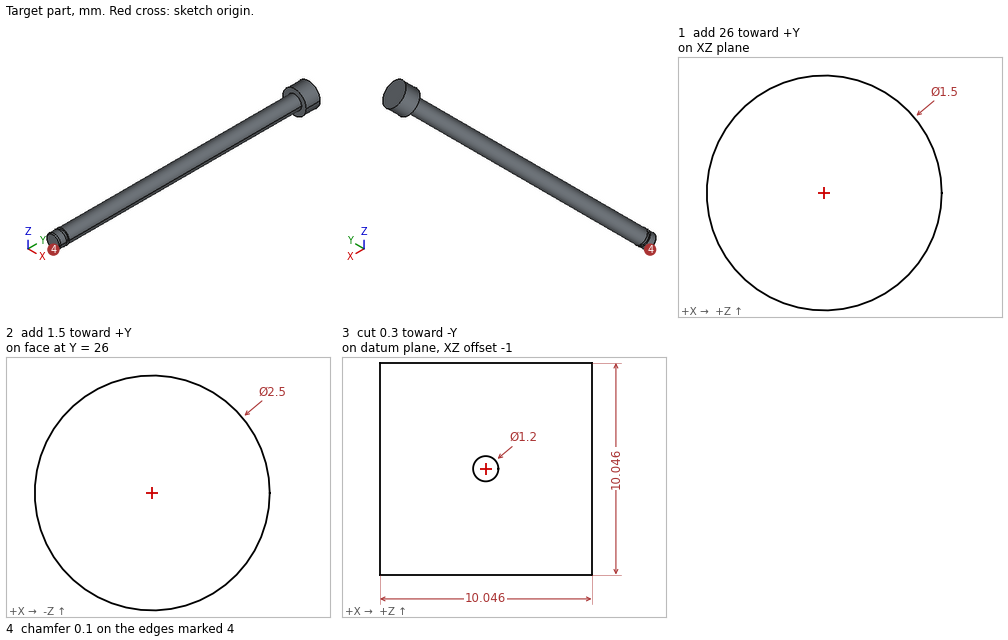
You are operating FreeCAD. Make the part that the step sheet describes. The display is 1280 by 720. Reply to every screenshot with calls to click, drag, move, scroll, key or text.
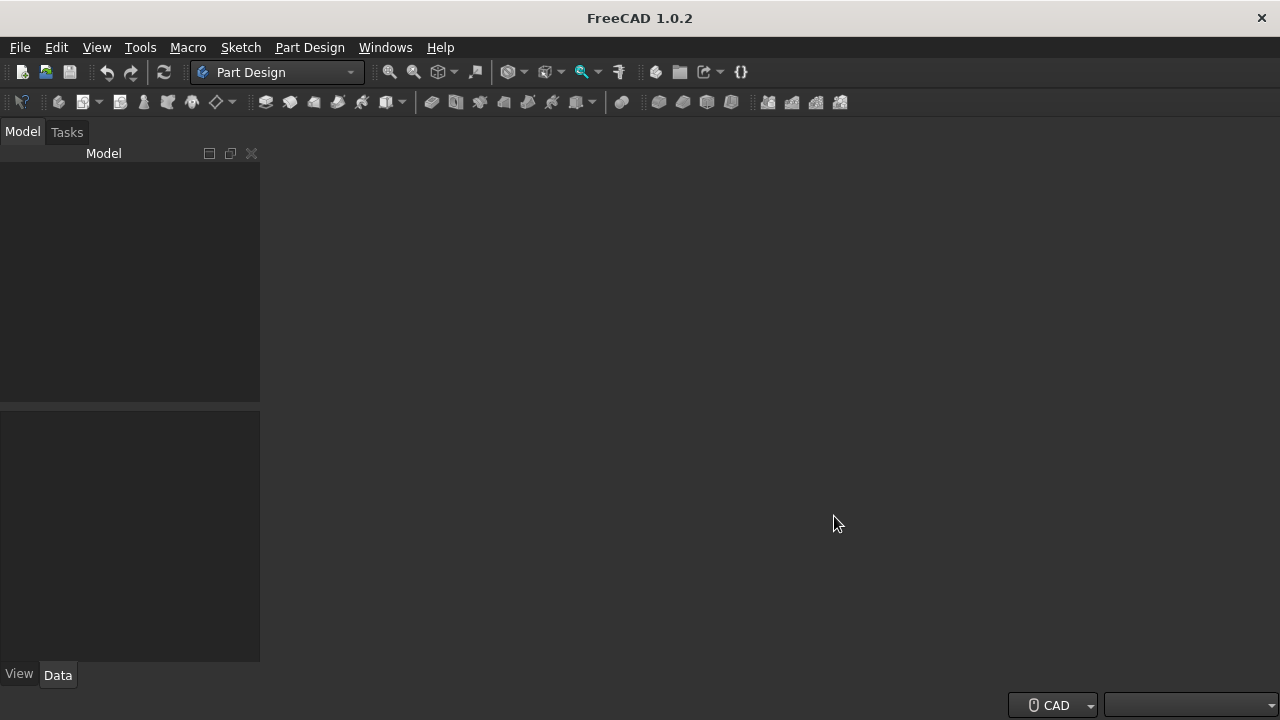
click(22, 72)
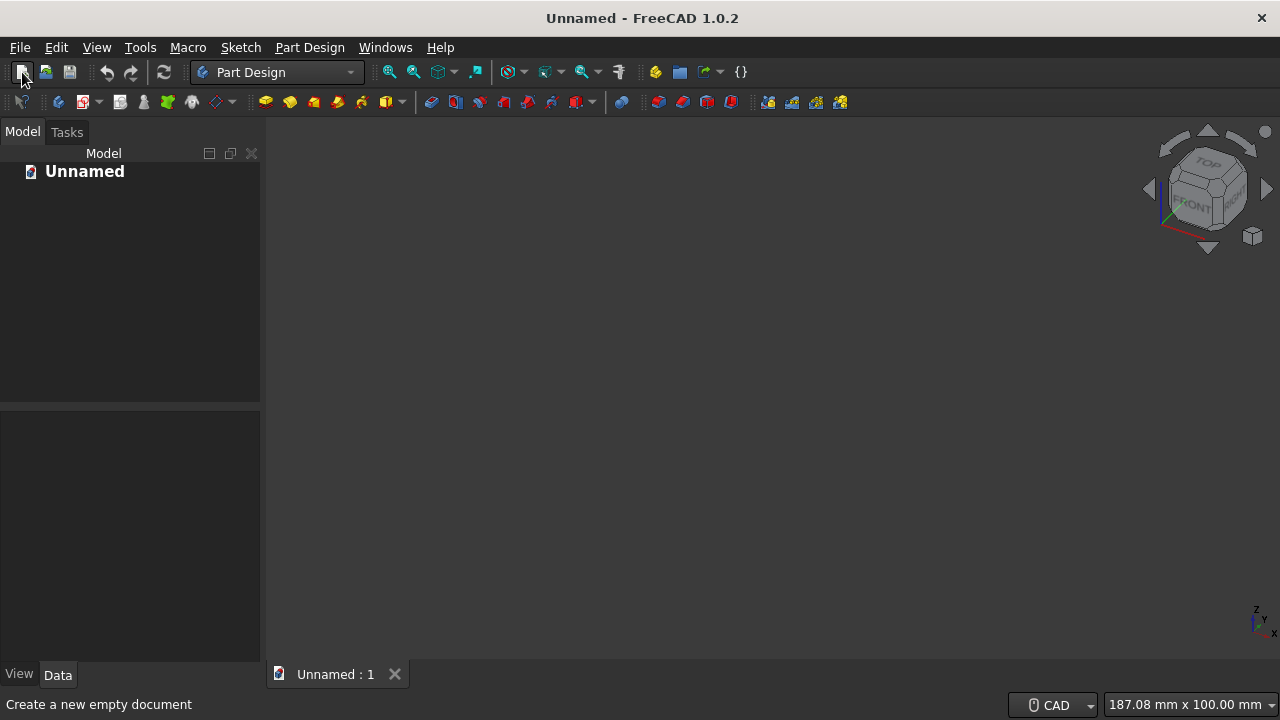
click(84, 102)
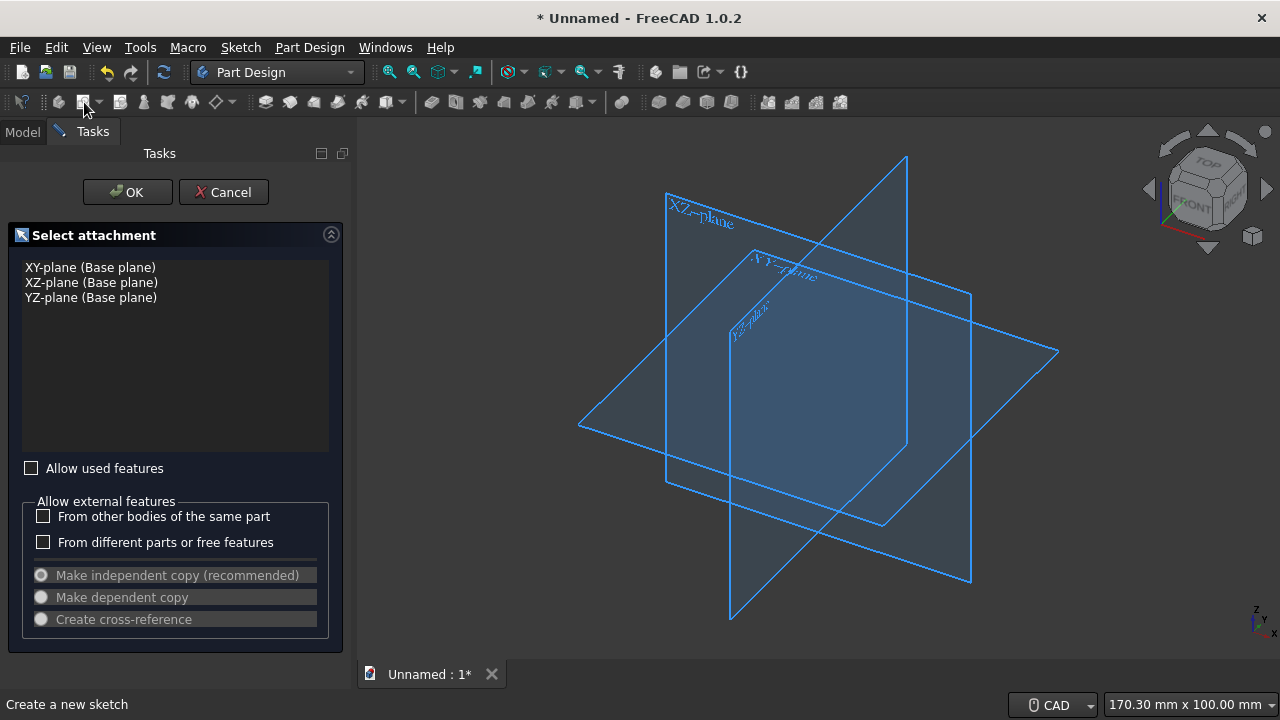
click(82, 282)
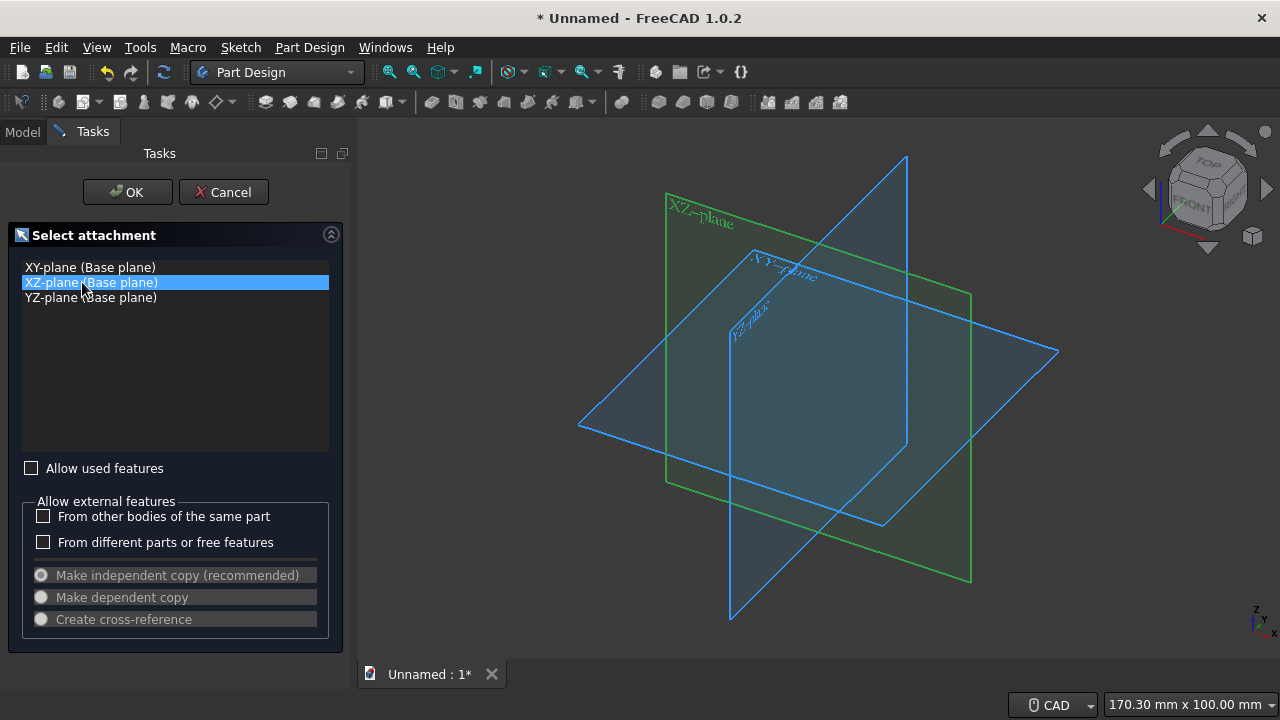
click(128, 192)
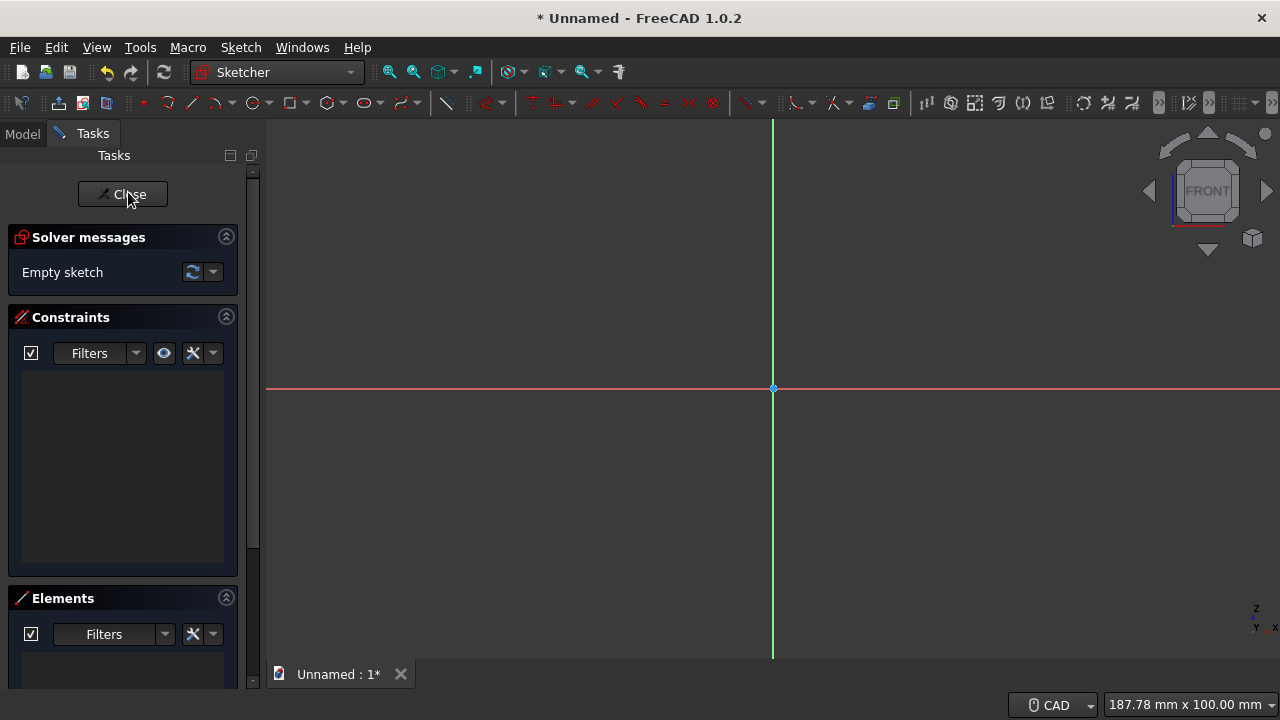
scroll(777, 389, up, 15)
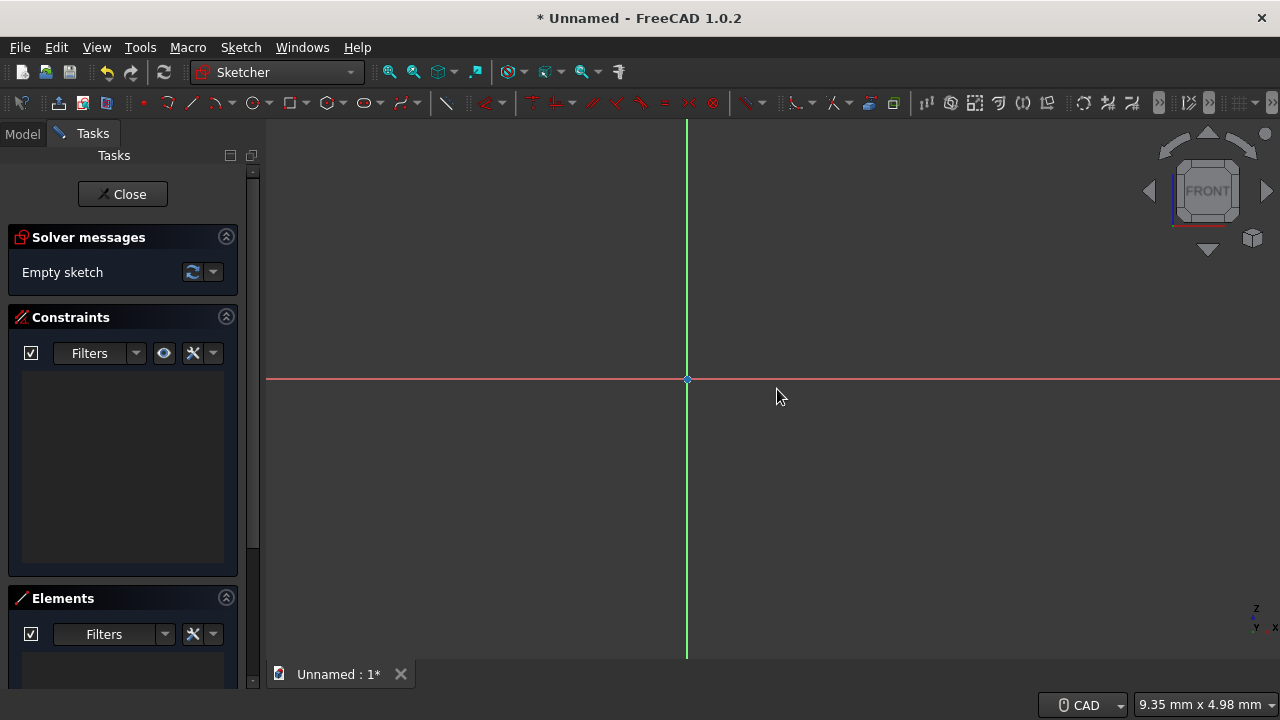
scroll(673, 372, up, 4)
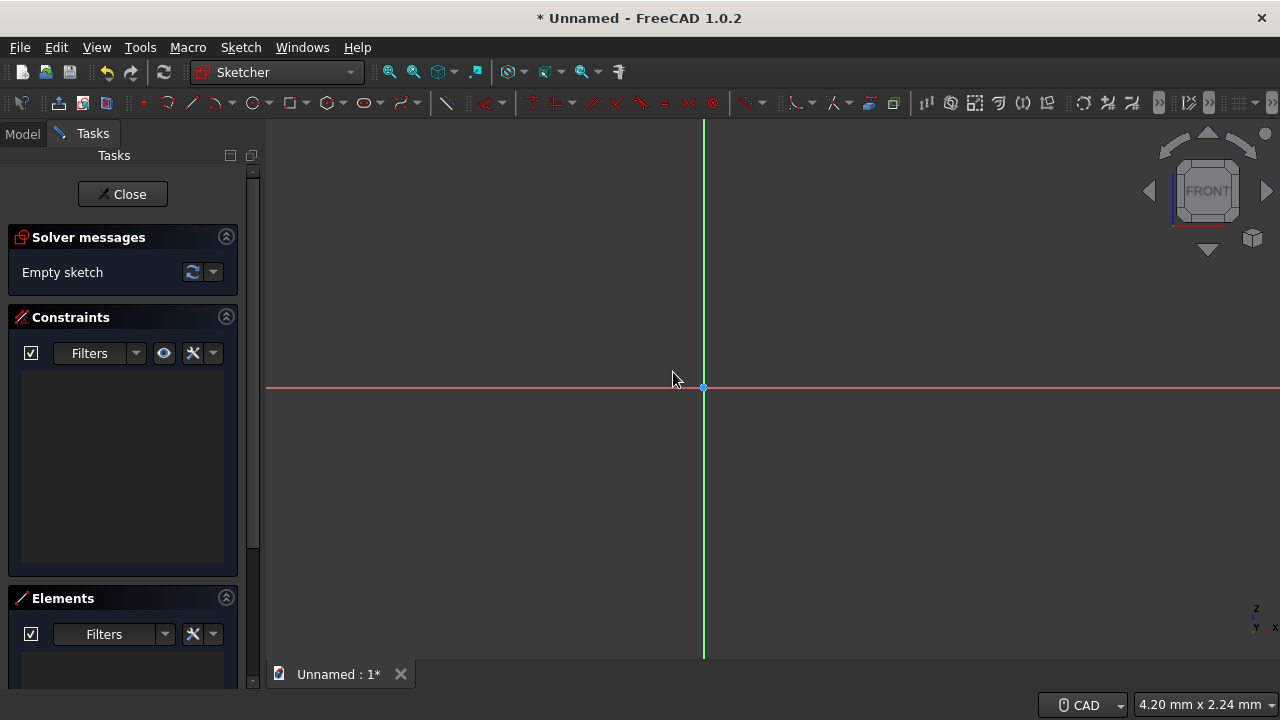
click(254, 104)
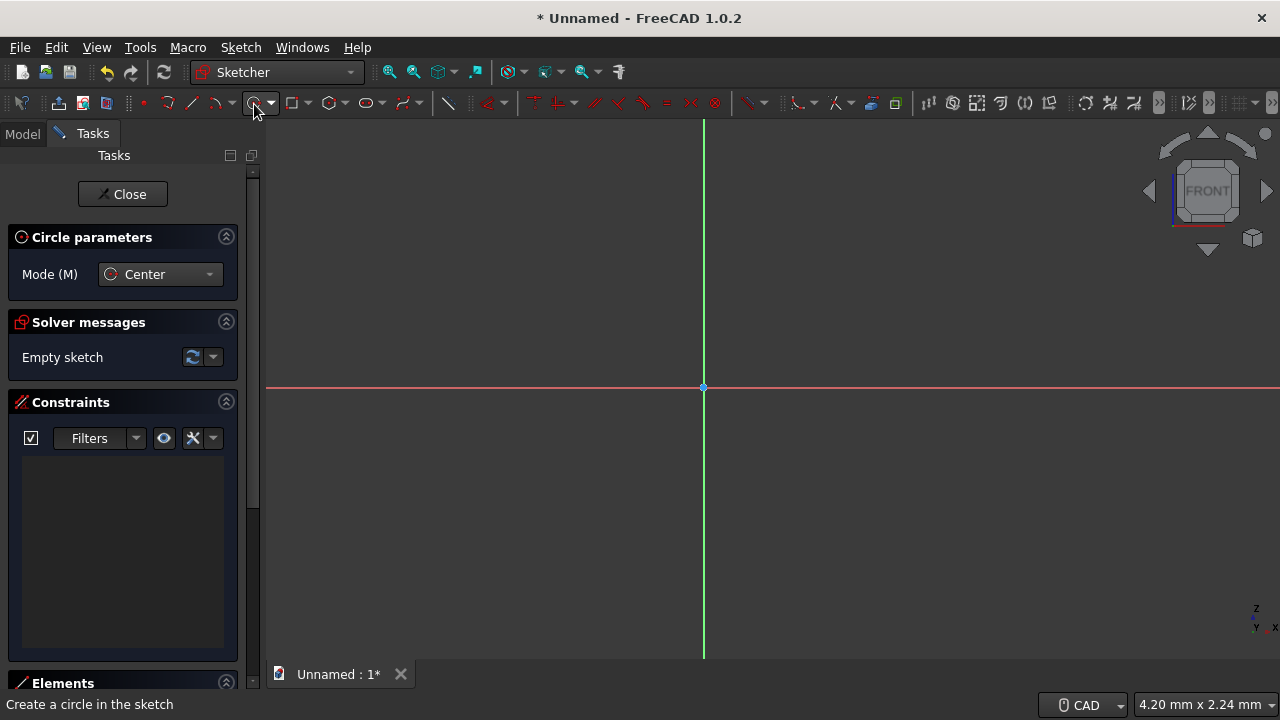
click(704, 388)
move(832, 260)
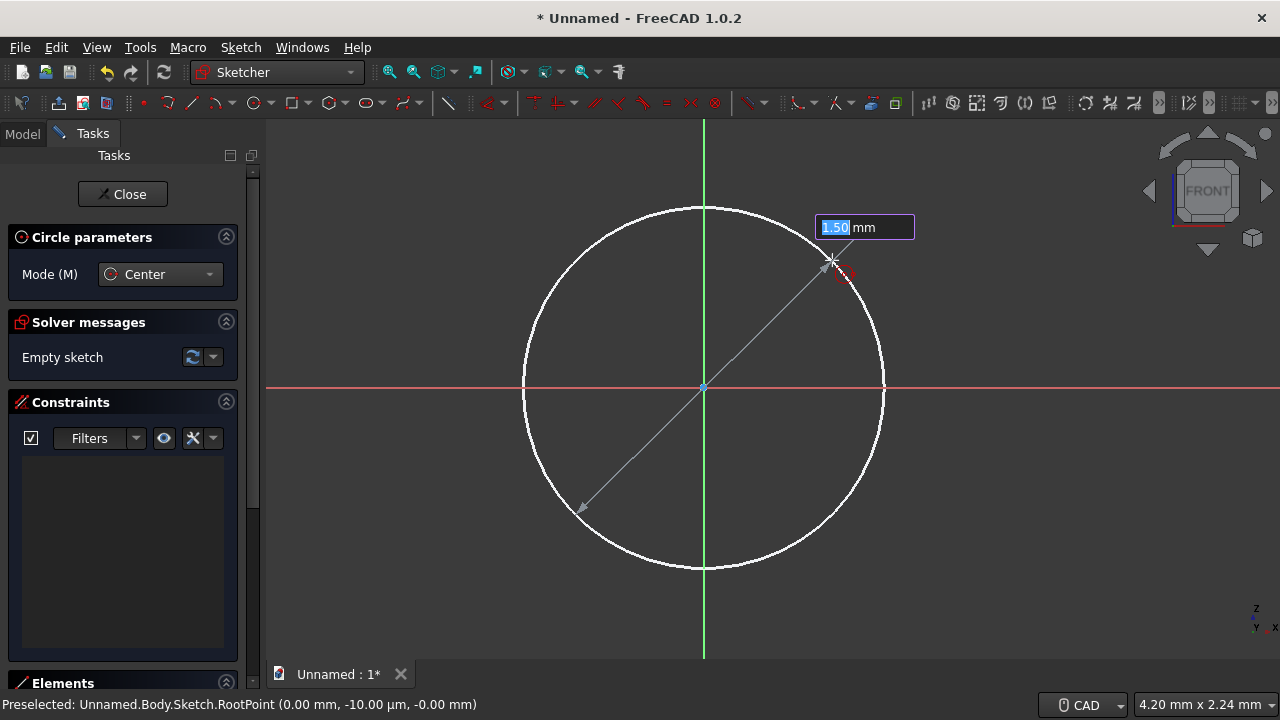
text(1.5)
key(Return)
key(Escape)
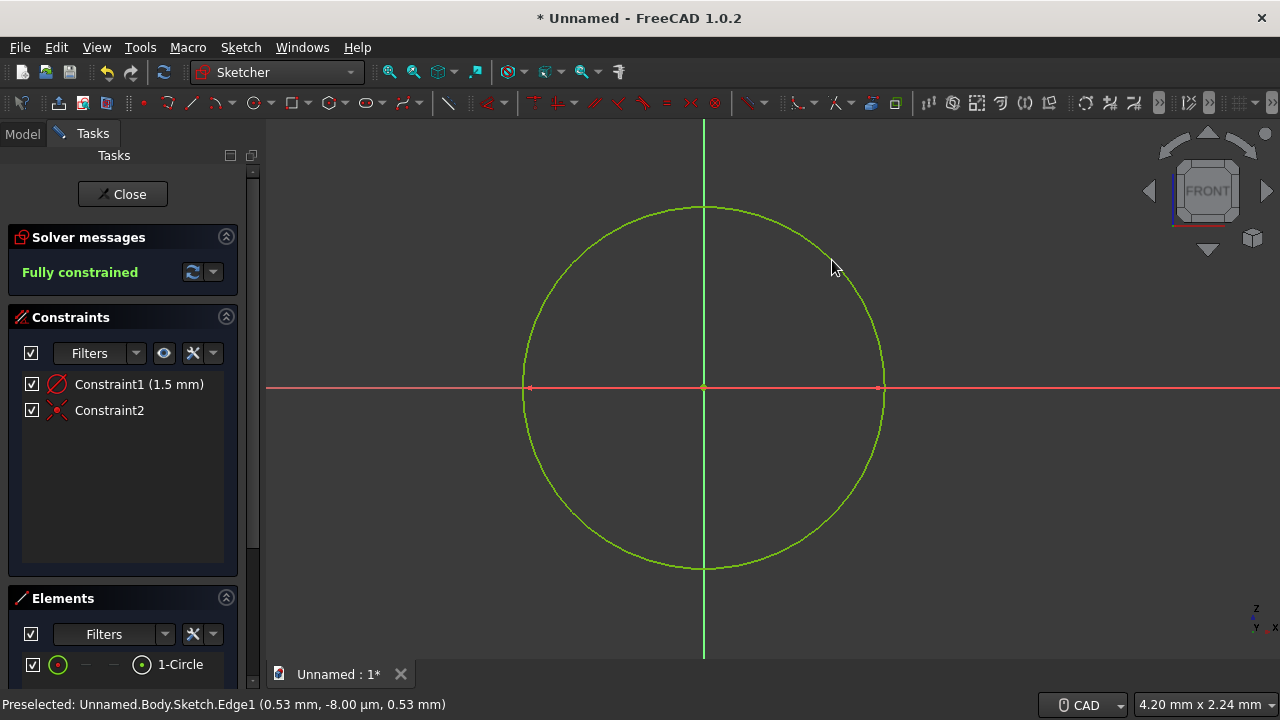
click(123, 194)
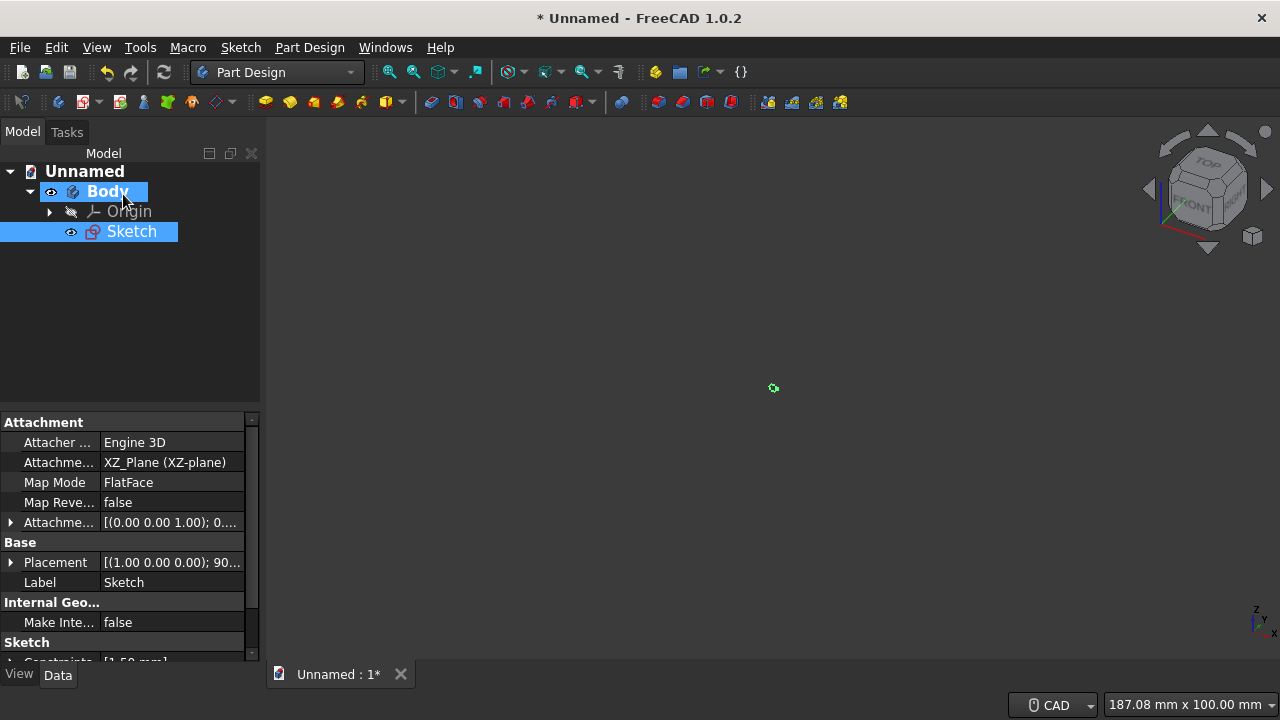
click(266, 102)